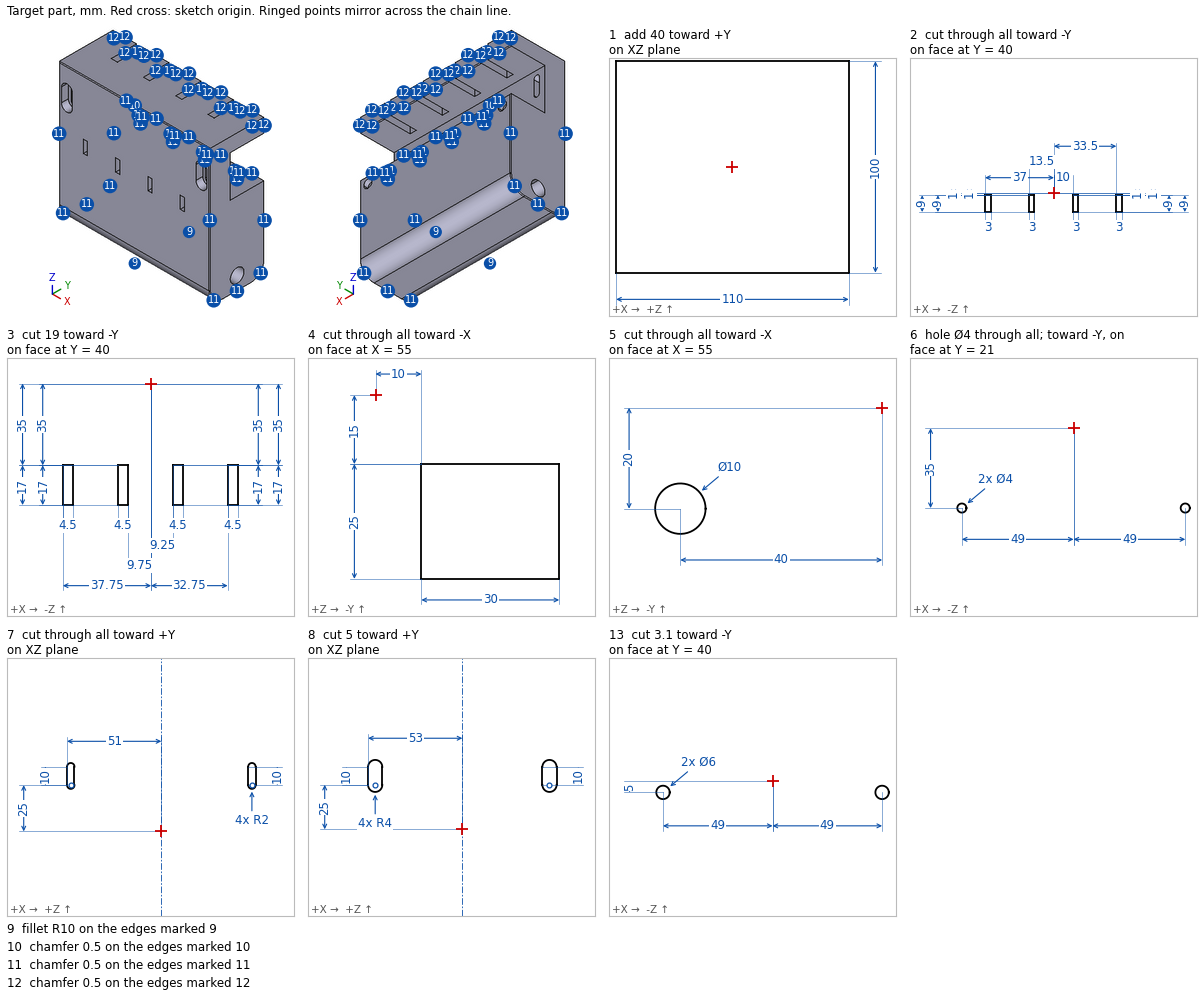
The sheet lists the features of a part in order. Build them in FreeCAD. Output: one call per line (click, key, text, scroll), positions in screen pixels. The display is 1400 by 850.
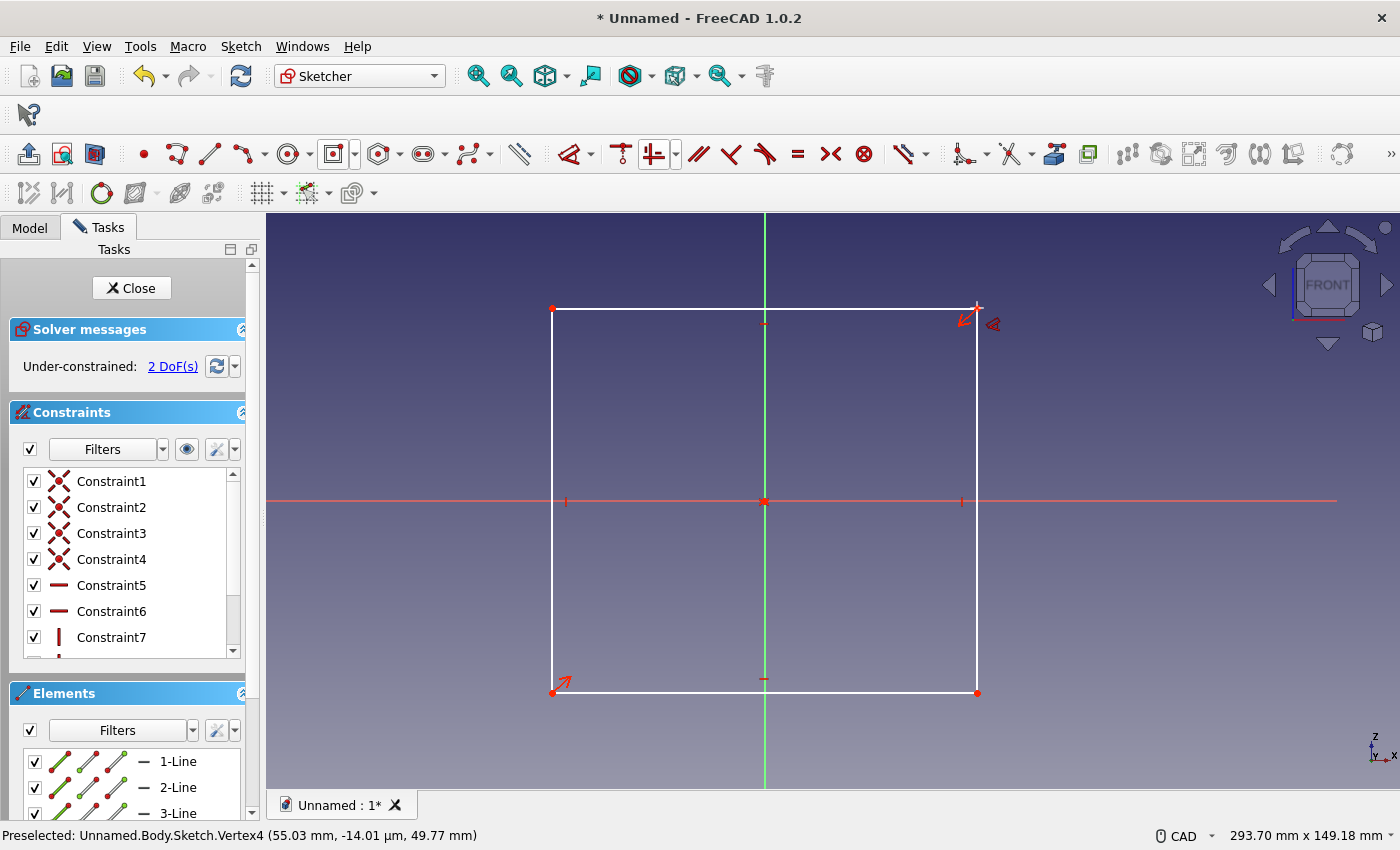
click(680, 693)
click(667, 727)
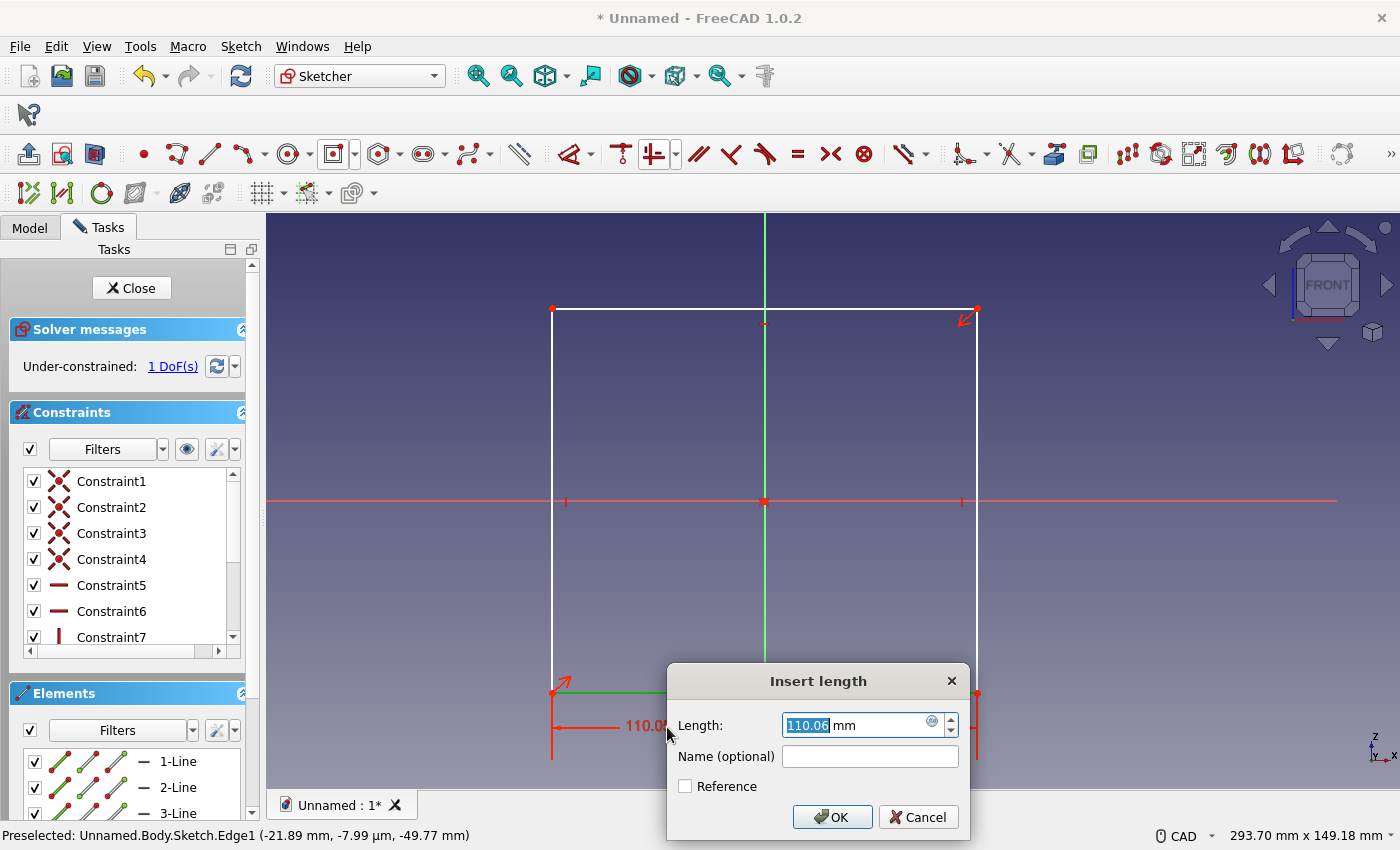
text(110)
key(Return)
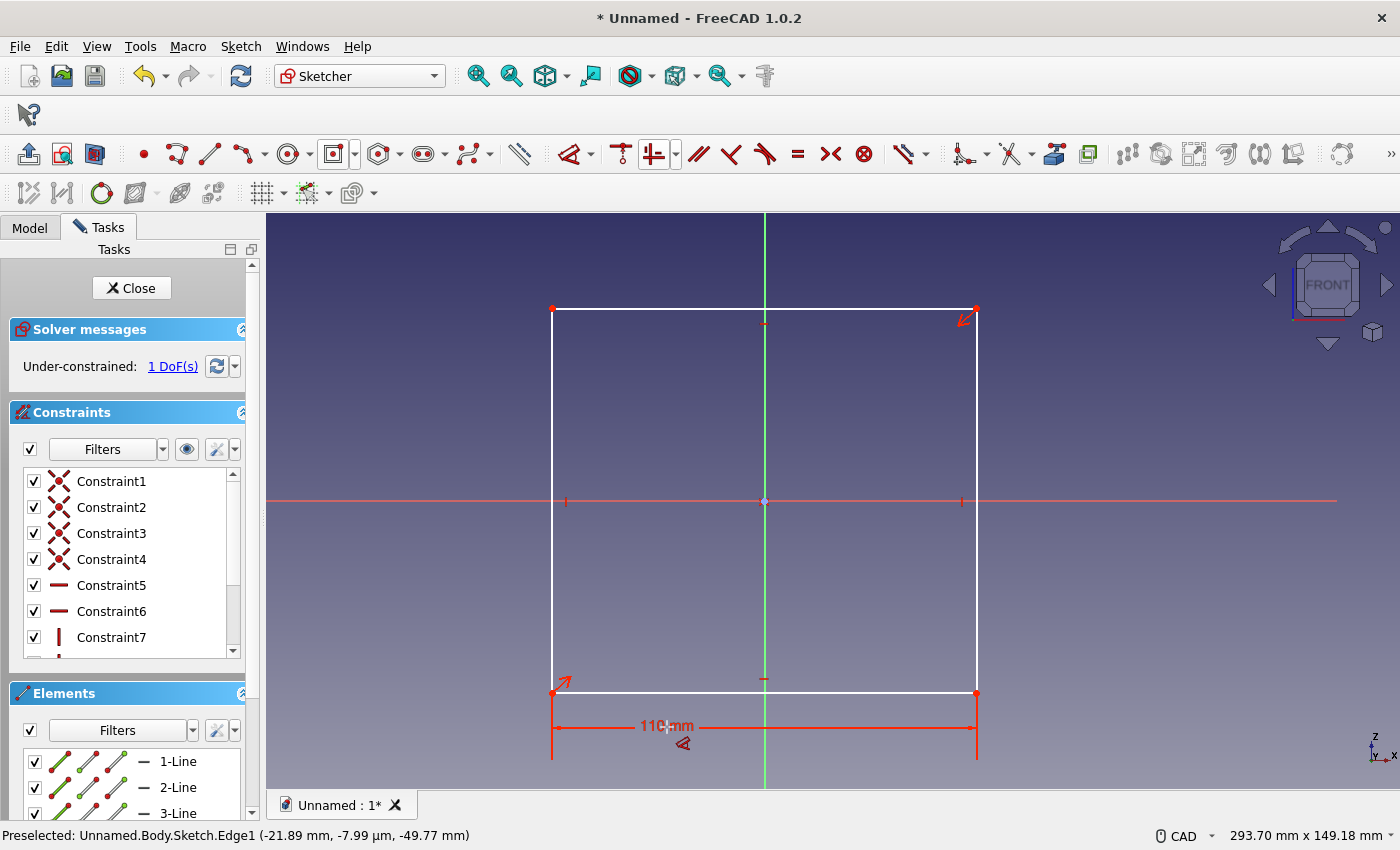
click(977, 578)
click(1011, 413)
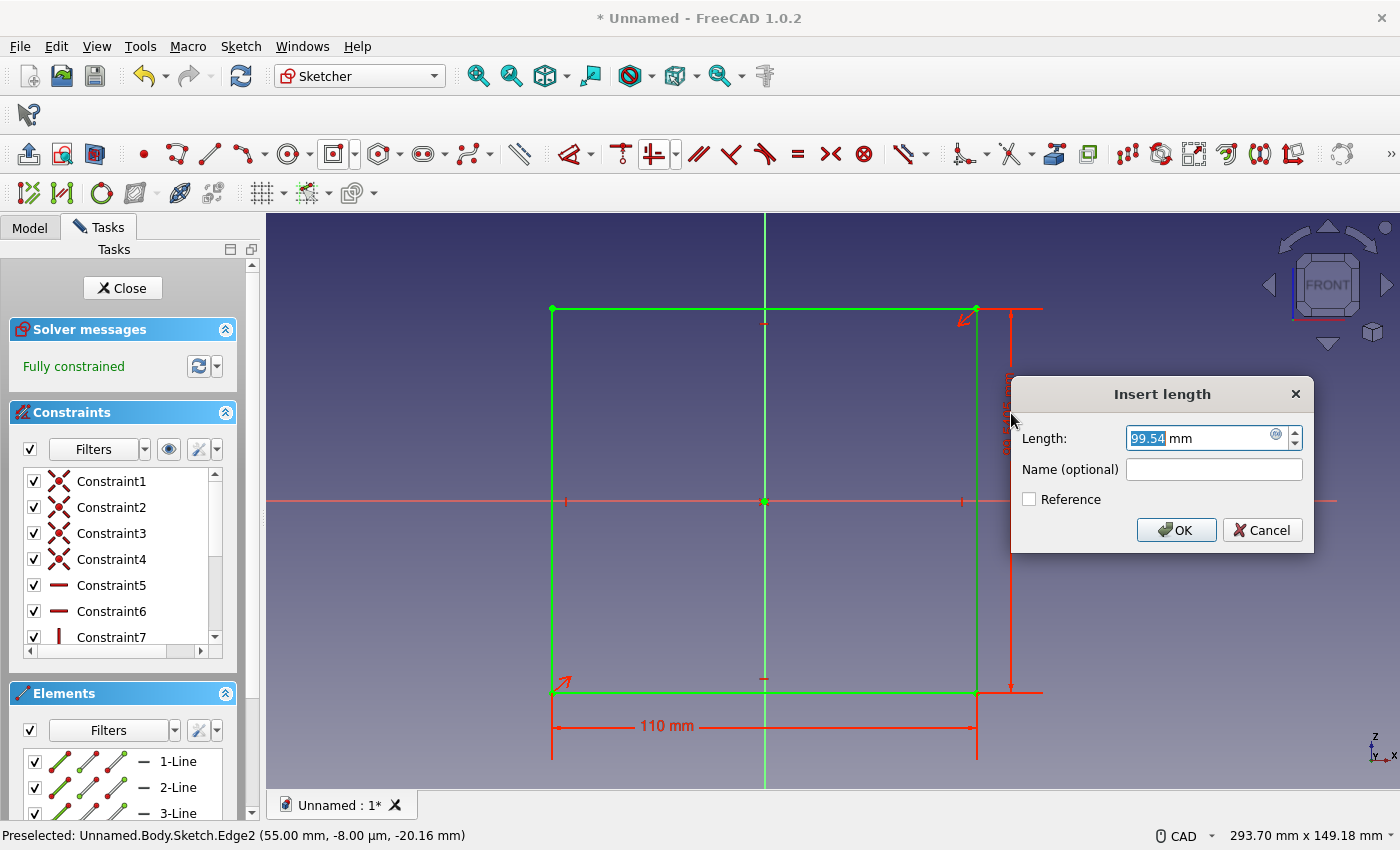
text(100)
key(Return)
key(Escape)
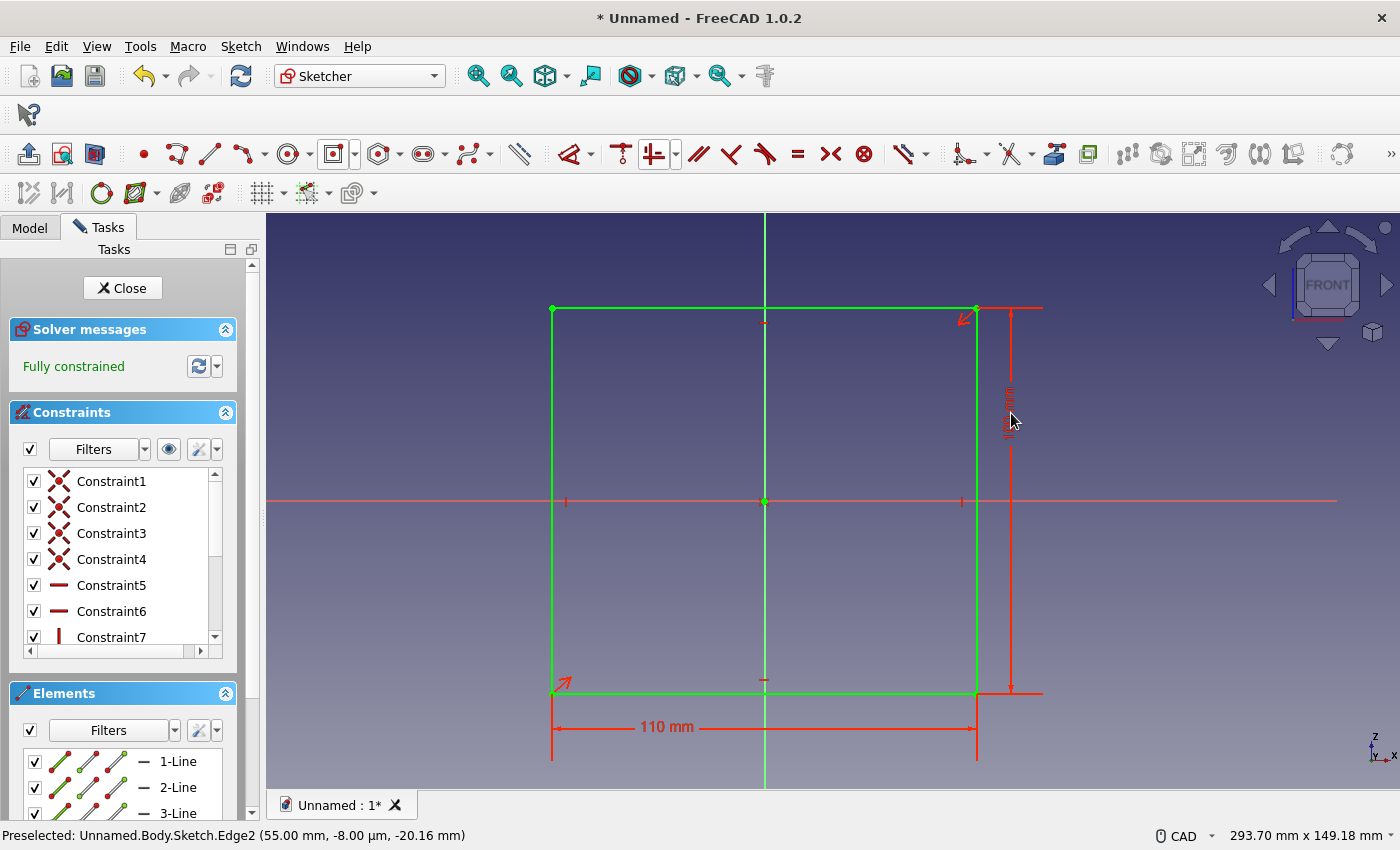
click(123, 288)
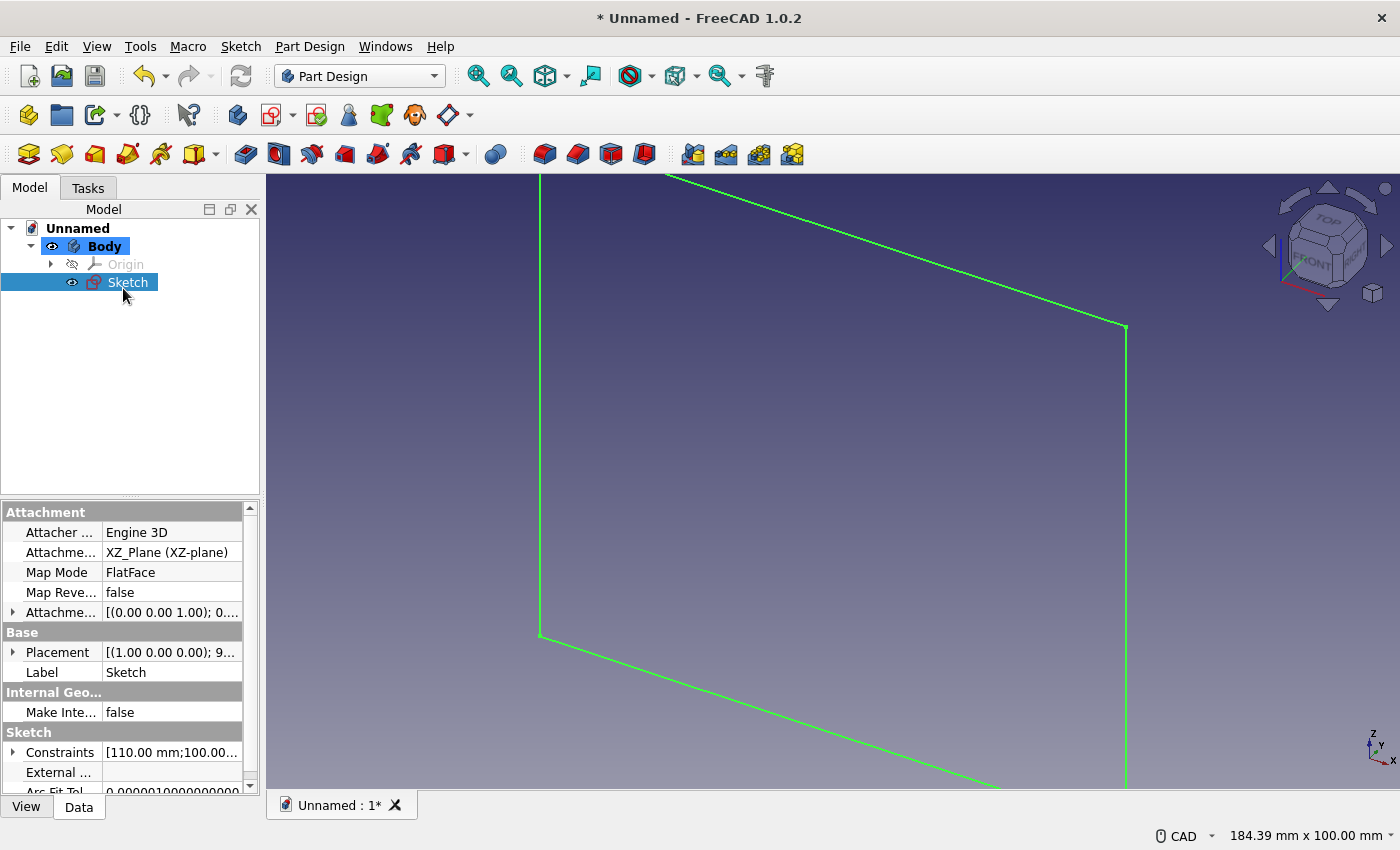
click(29, 154)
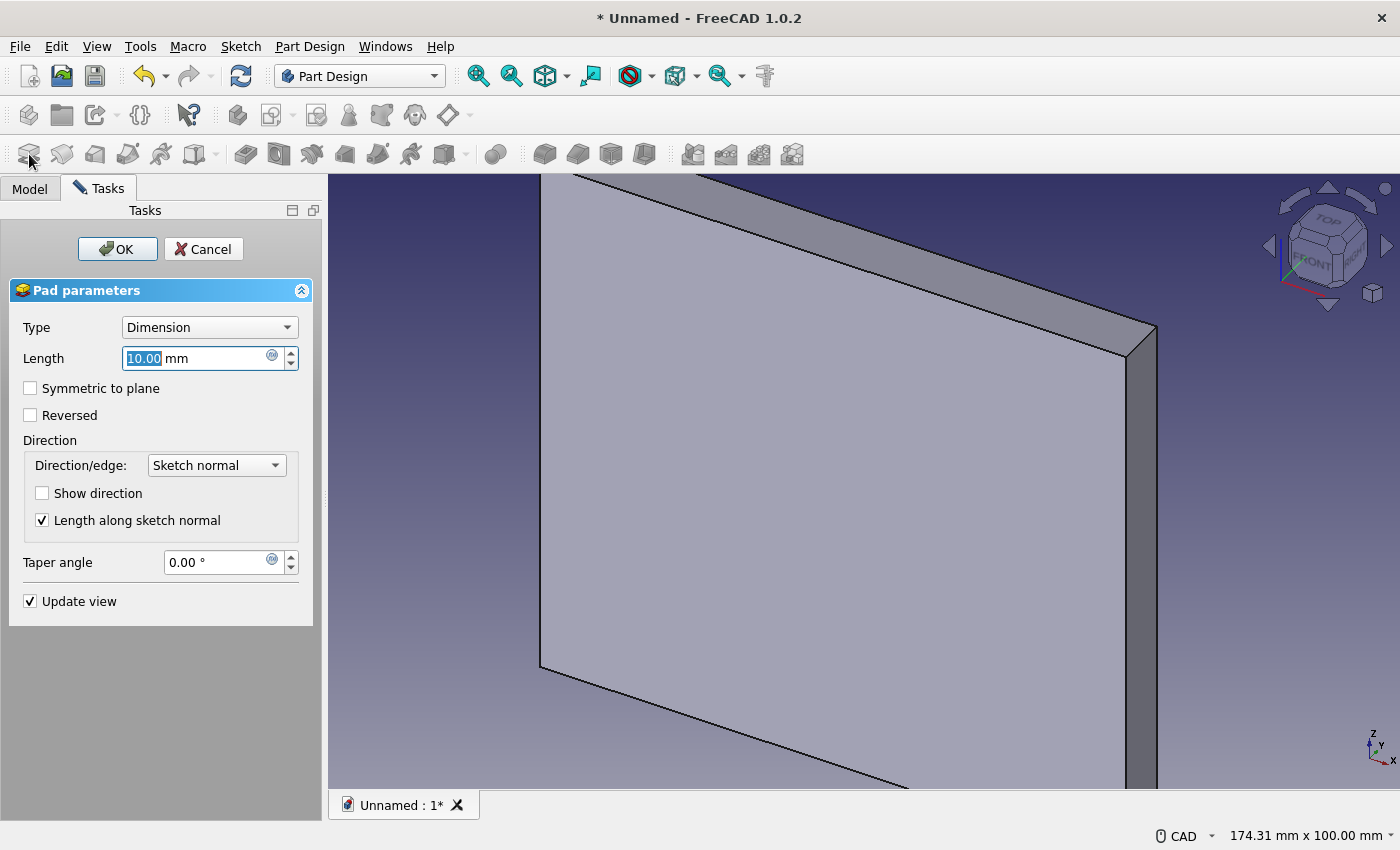
text(40)
key(Tab)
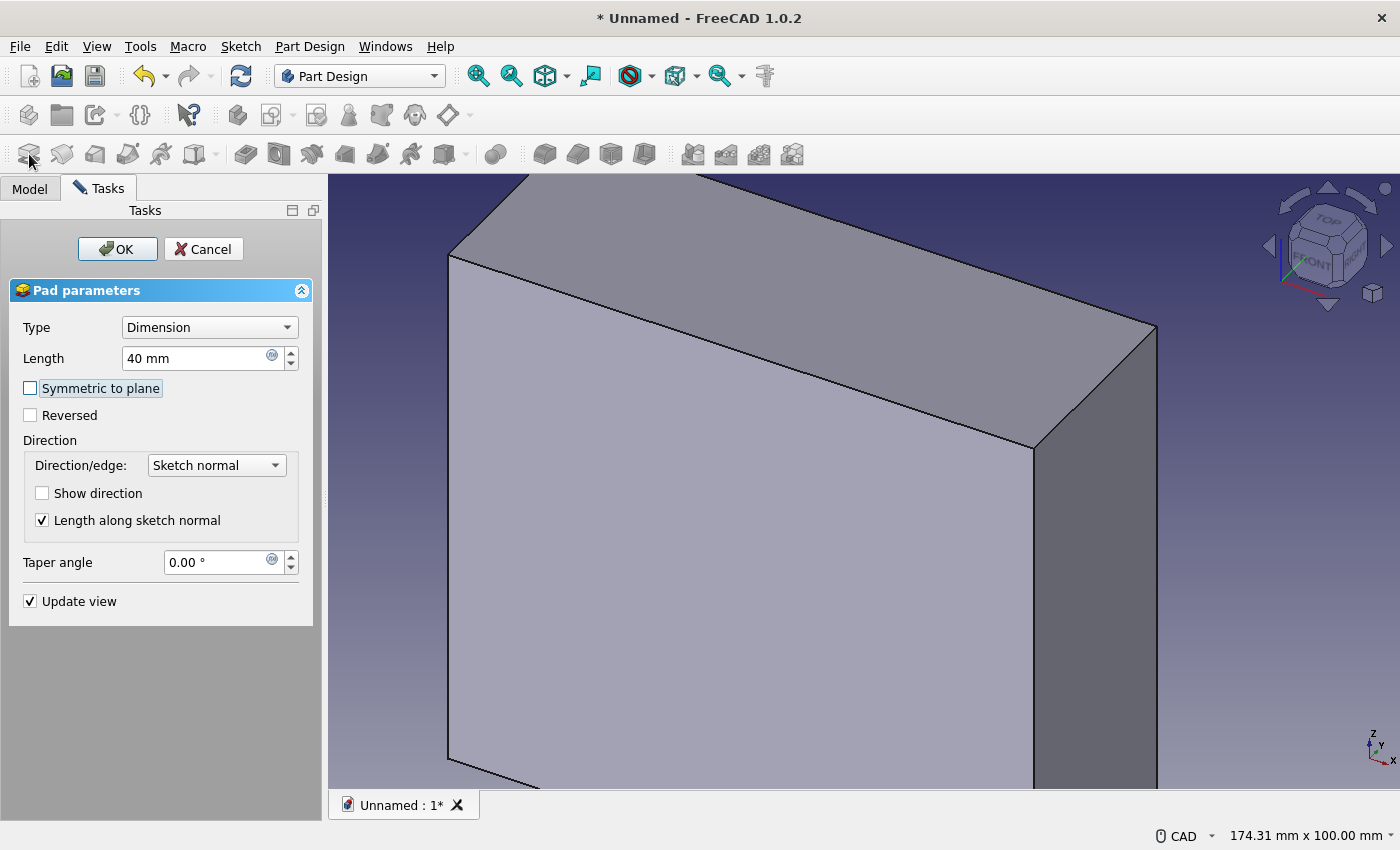
click(31, 415)